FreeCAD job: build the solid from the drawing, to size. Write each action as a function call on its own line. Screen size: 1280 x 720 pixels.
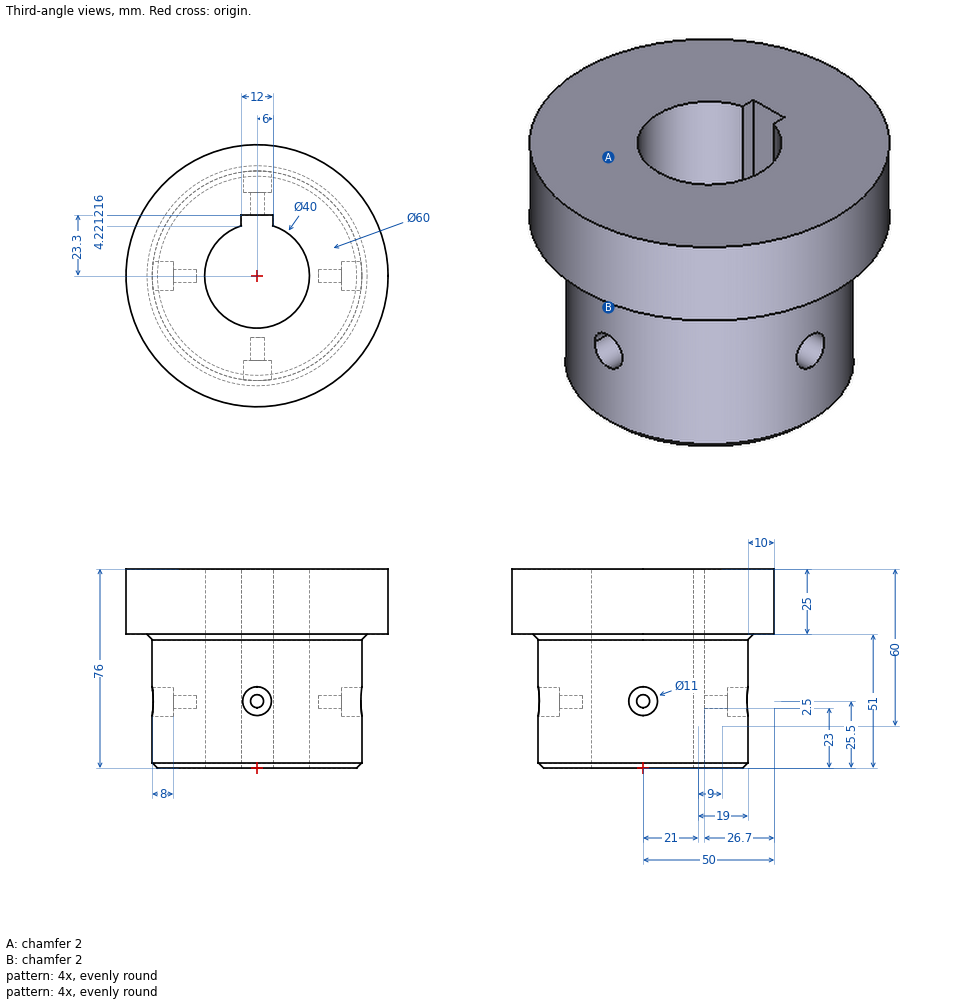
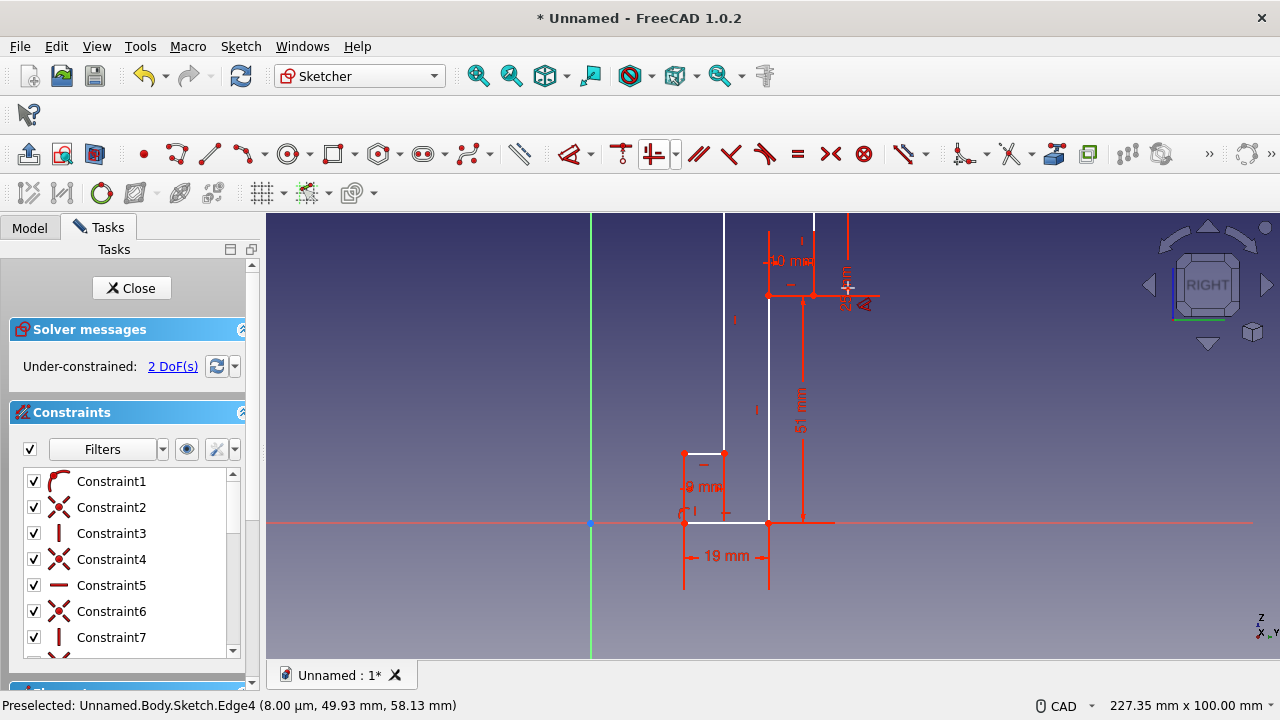
click(724, 265)
click(690, 347)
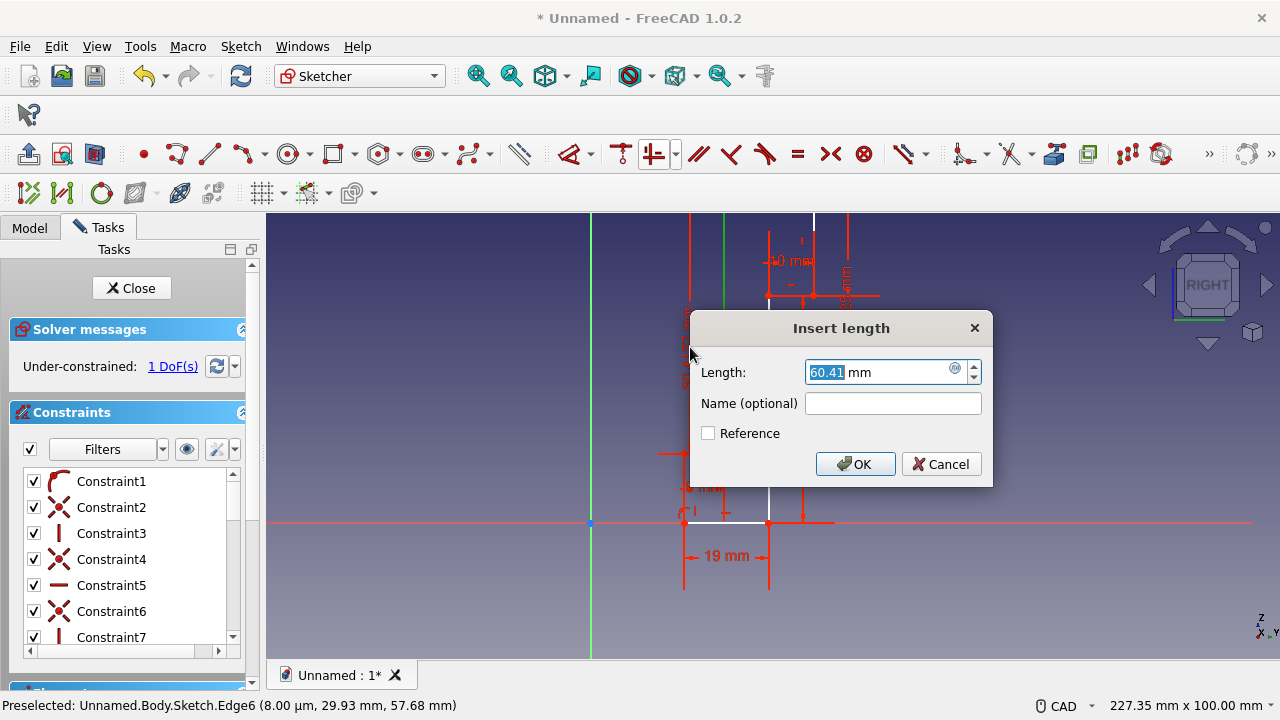
text(60)
key(Return)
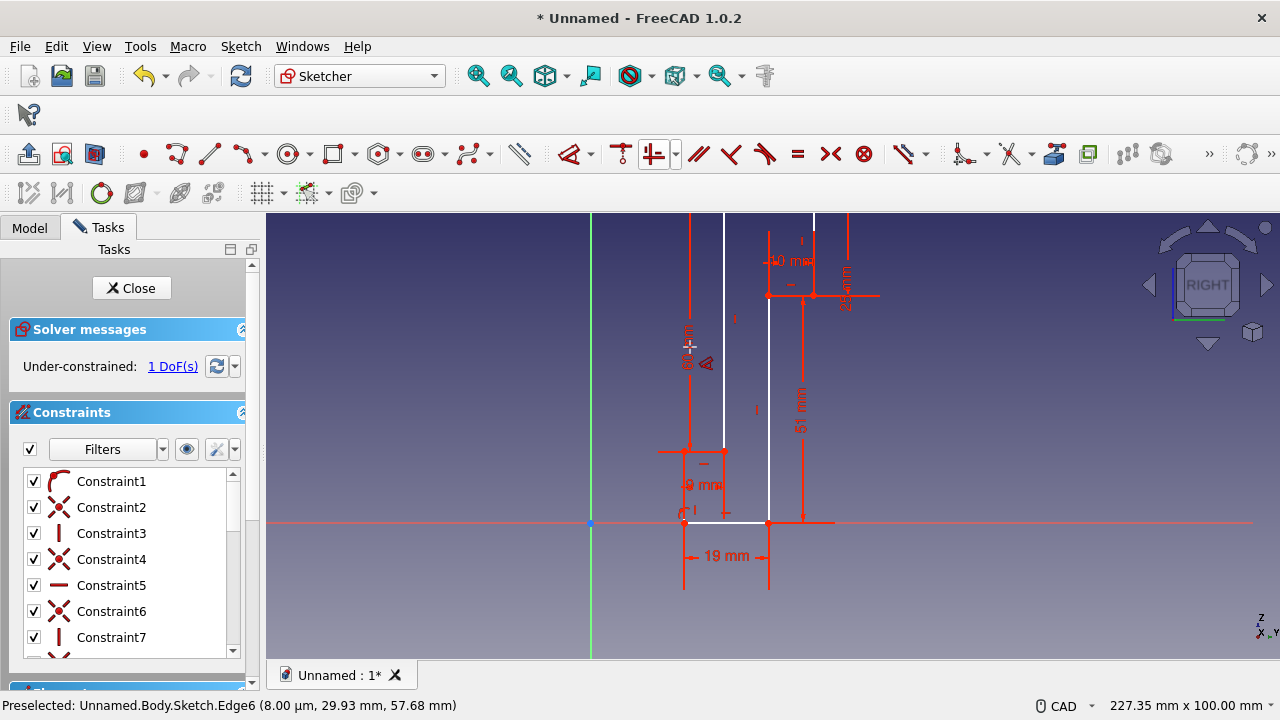
click(684, 523)
click(638, 557)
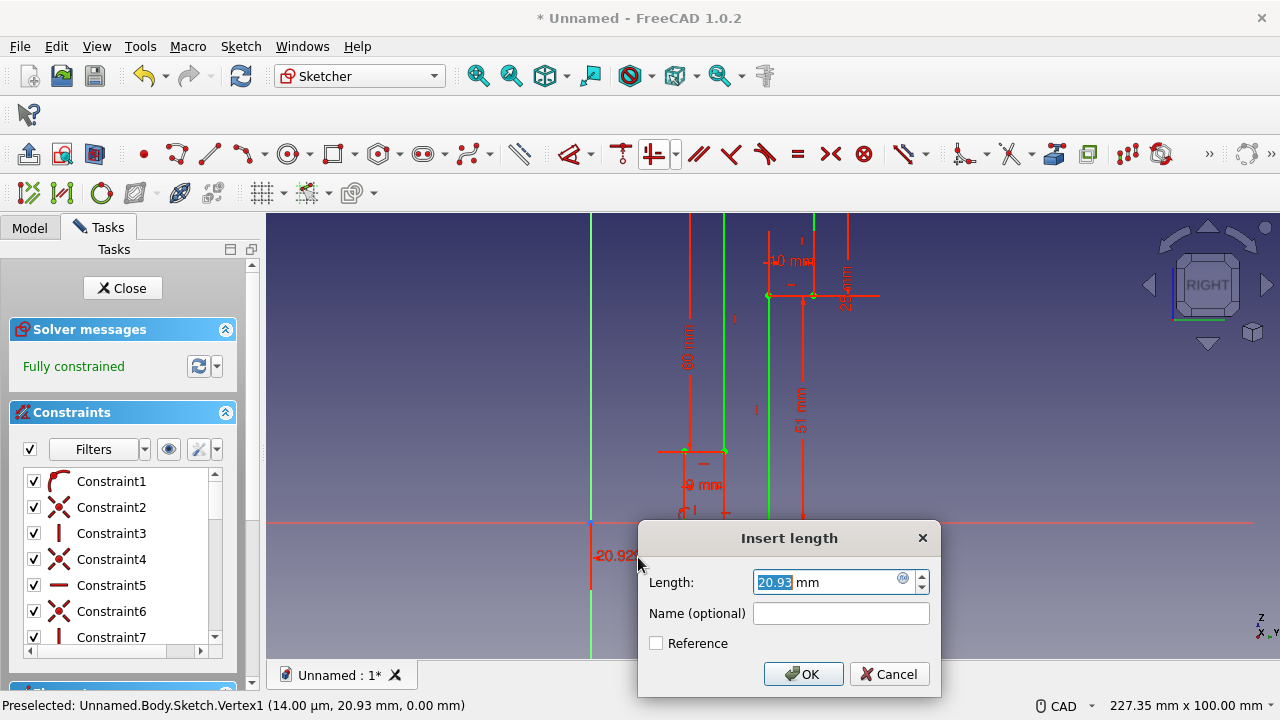
text(21)
key(Return)
key(Escape)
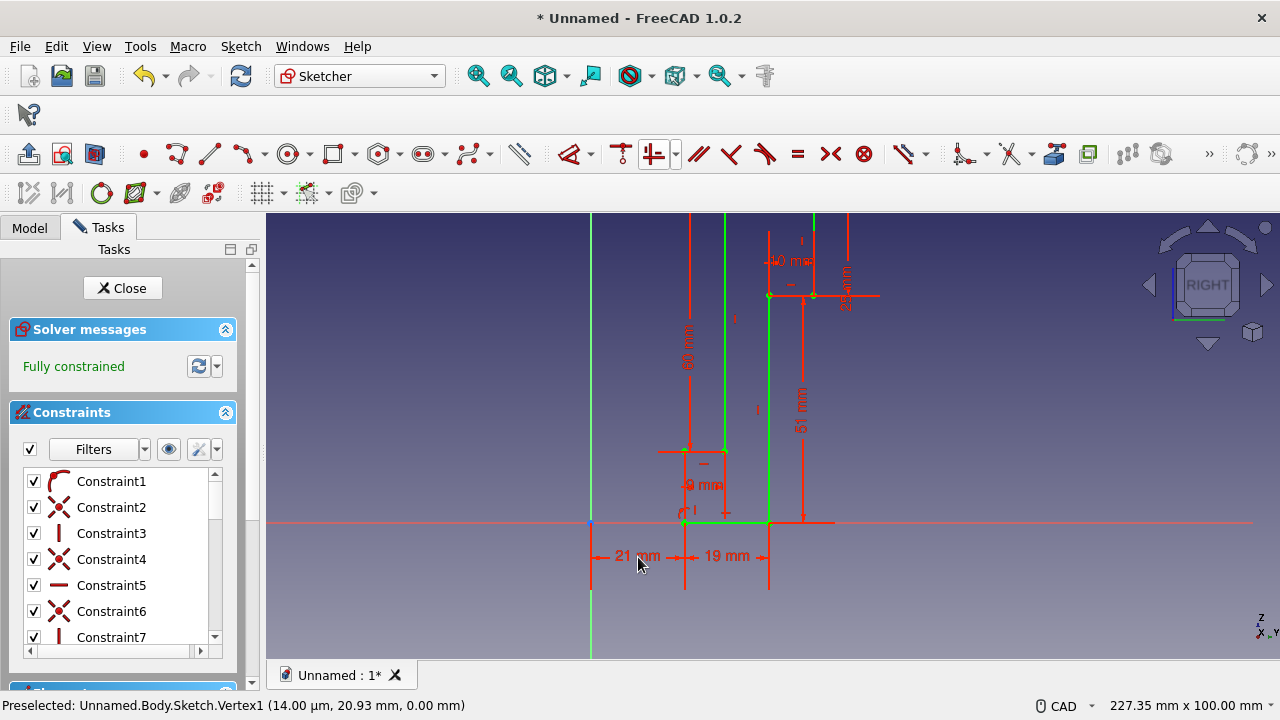
click(123, 288)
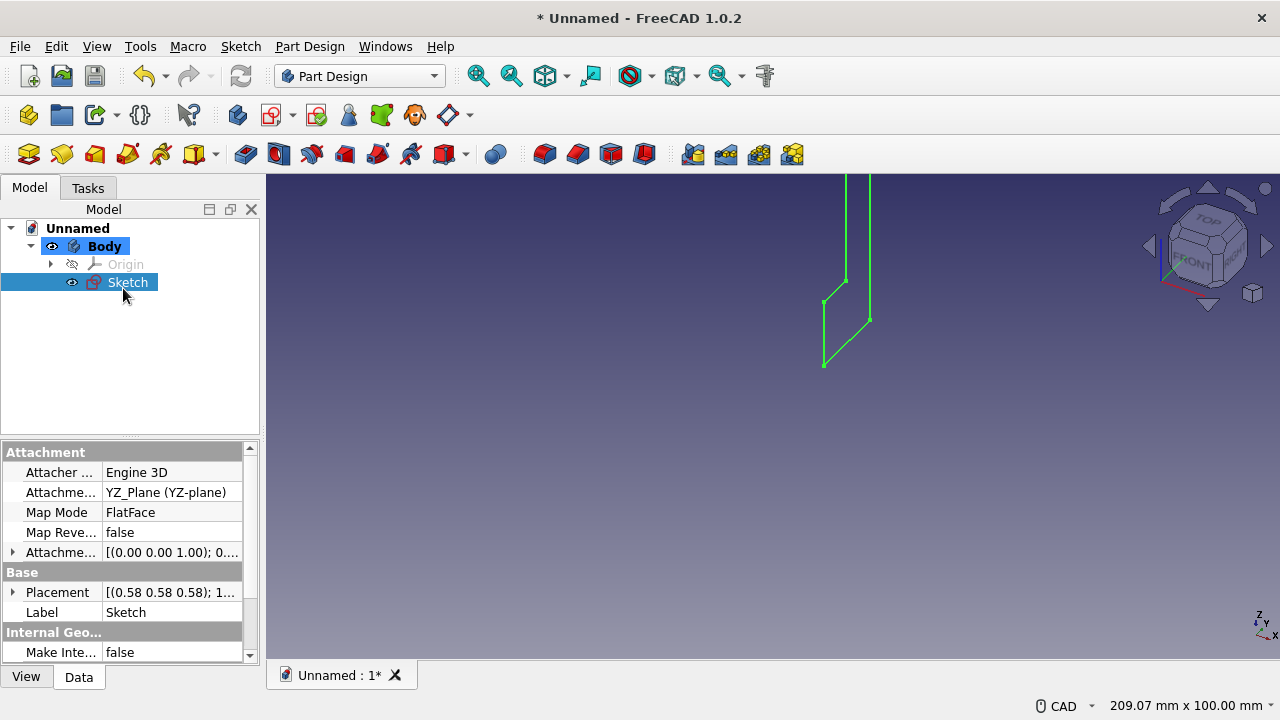
click(62, 154)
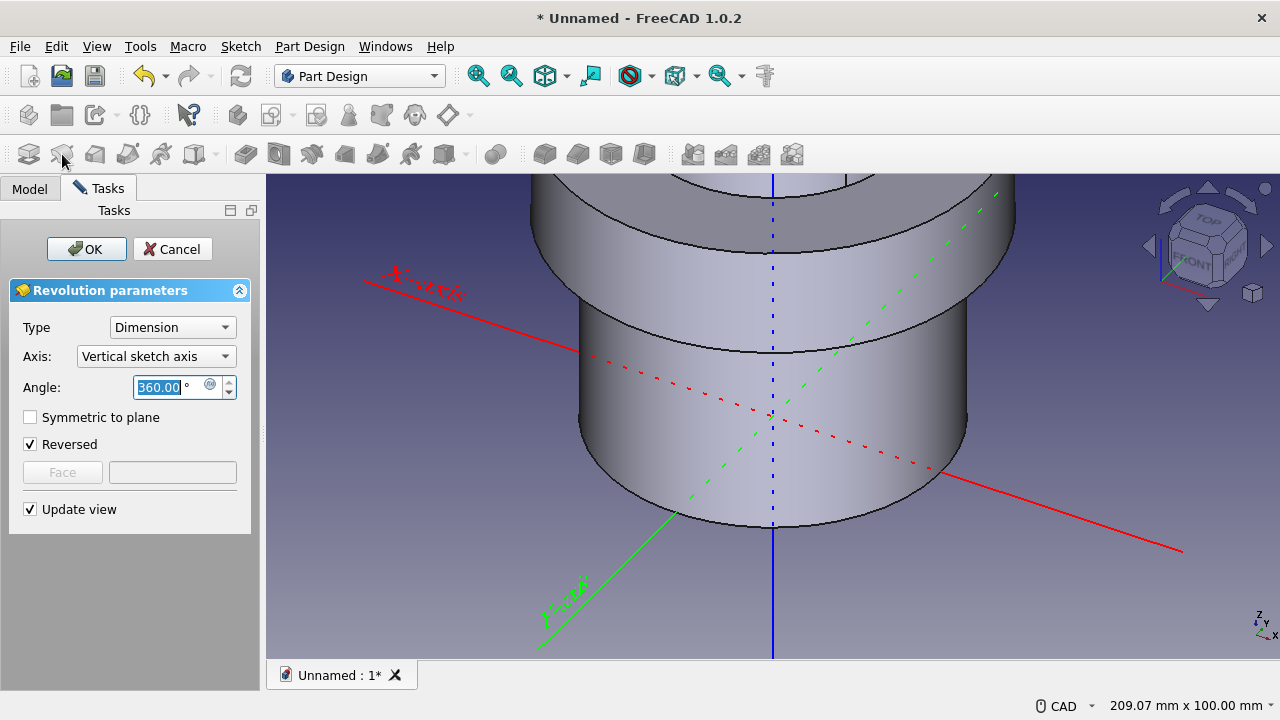
click(87, 249)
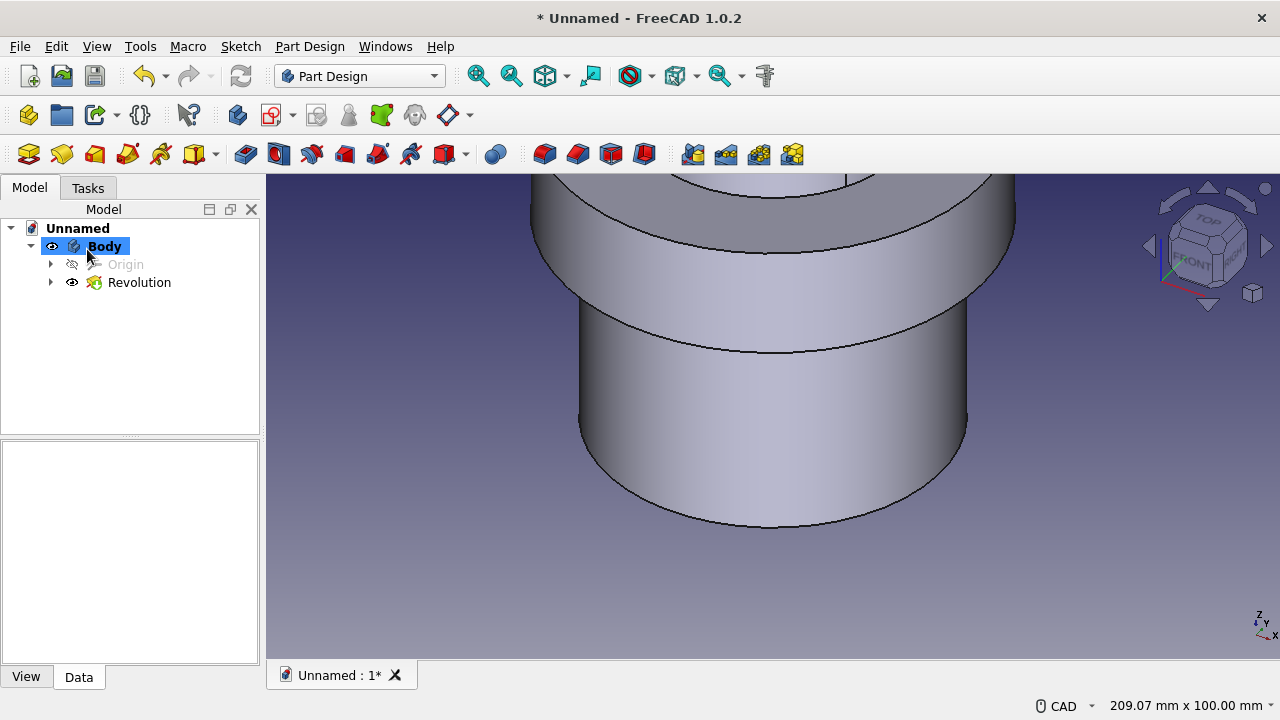
key(v)
key(f)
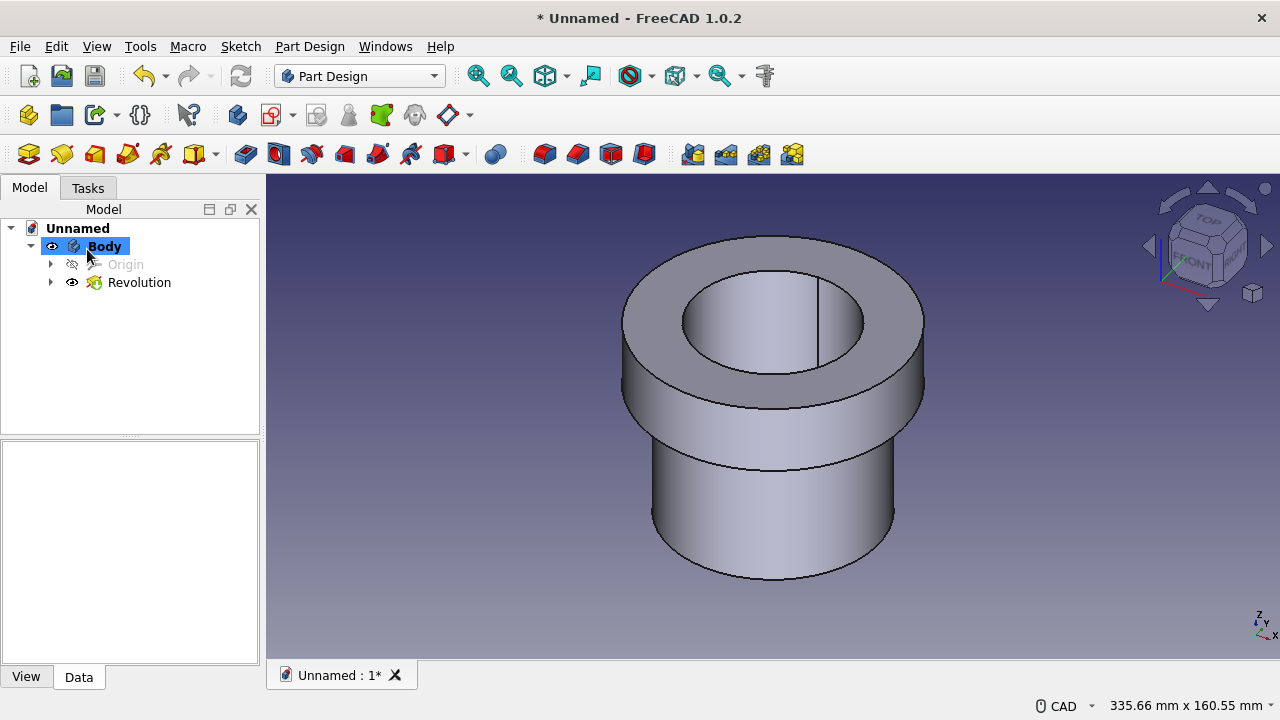
key(0)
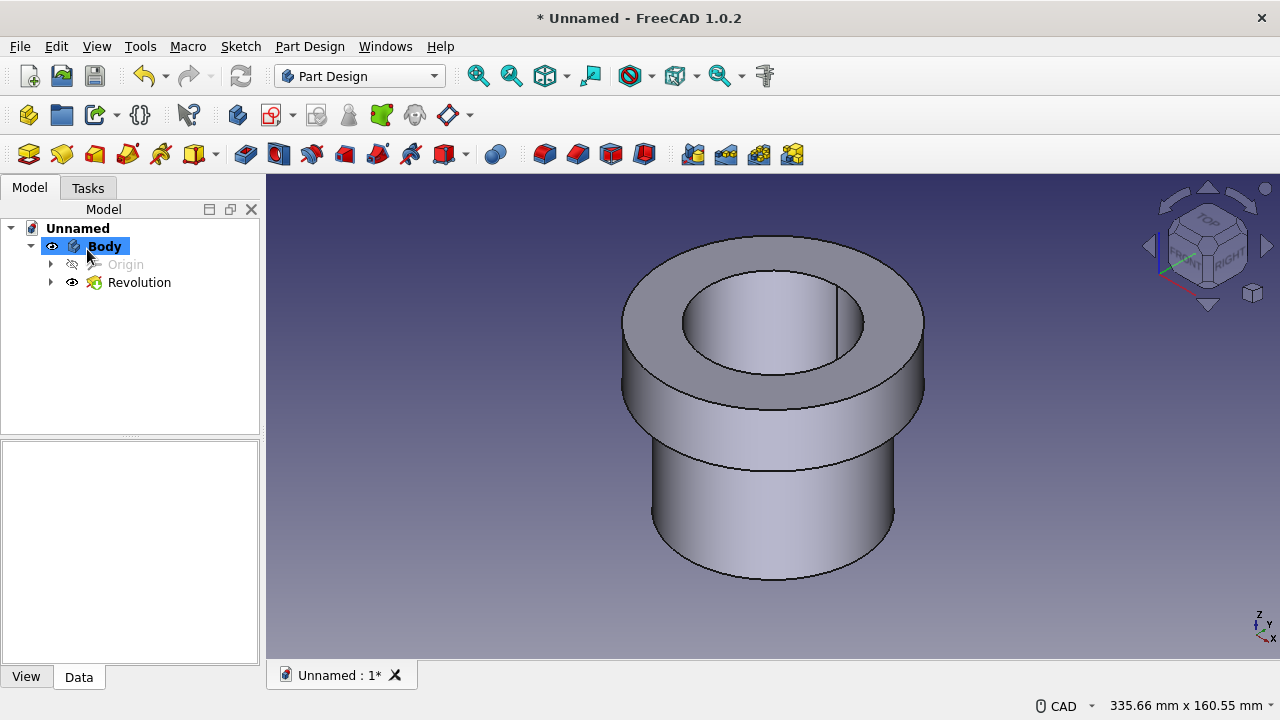
key(2)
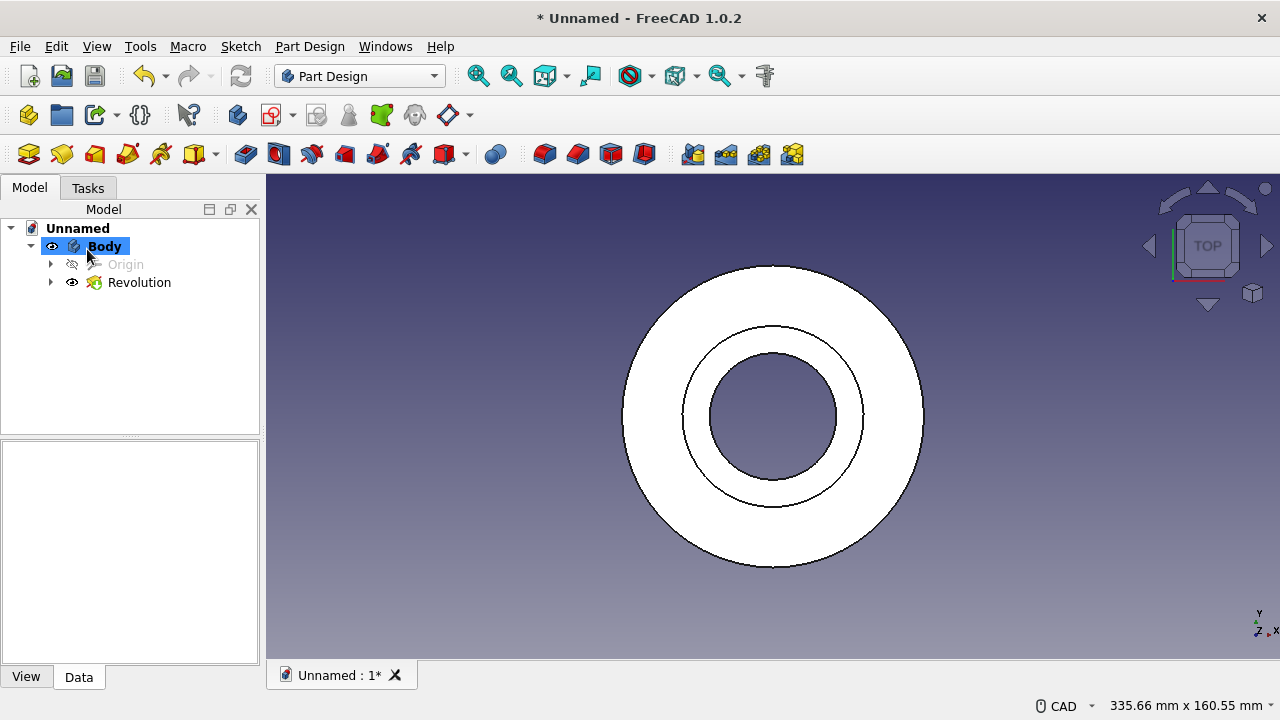
key(1)